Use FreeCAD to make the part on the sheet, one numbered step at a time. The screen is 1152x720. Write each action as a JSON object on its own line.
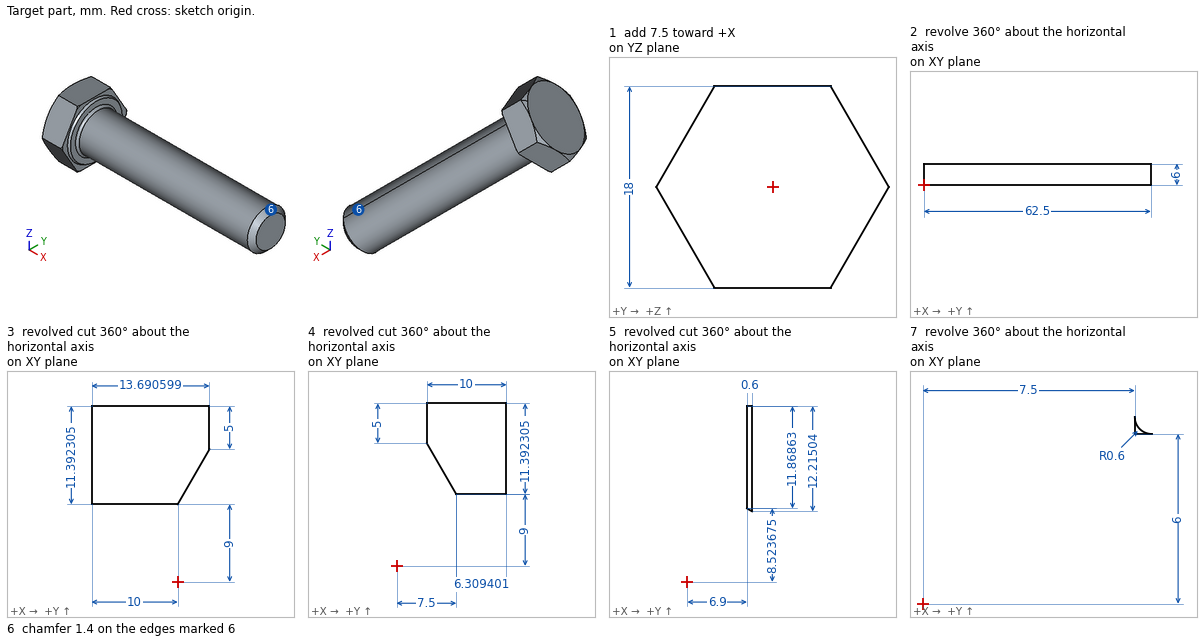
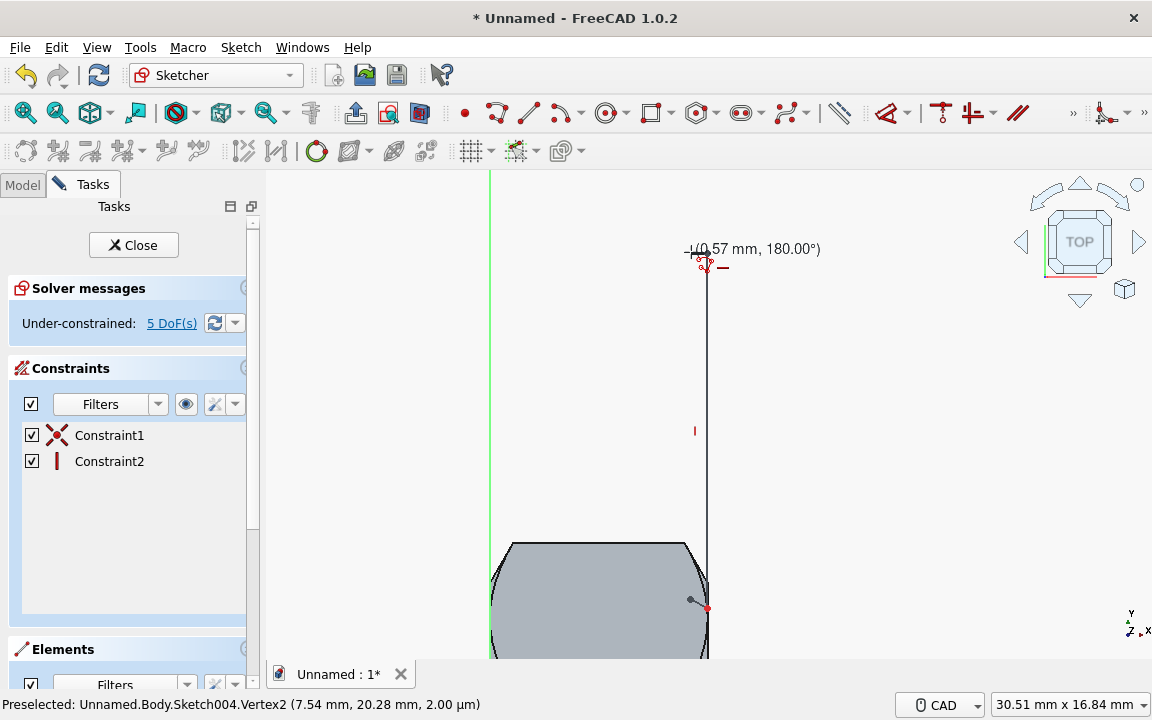
{"action": "left_click", "coordinate": [690, 252]}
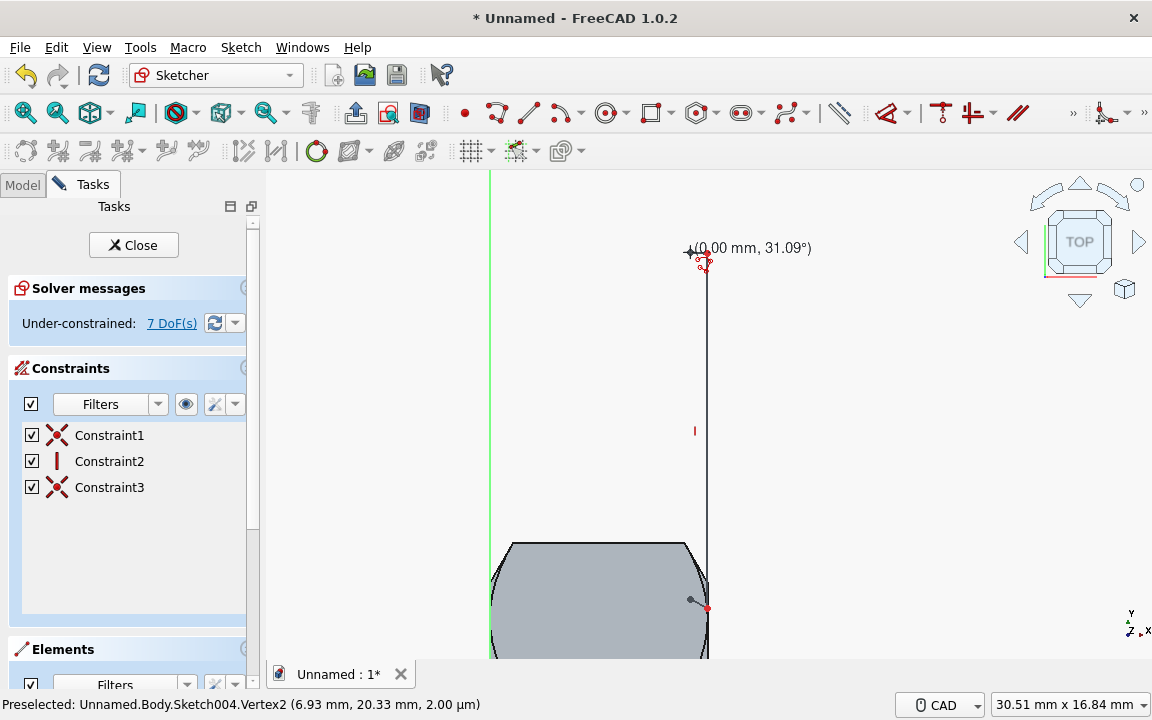
{"action": "scroll", "coordinate": [690, 597], "scroll_direction": "up", "scroll_amount": 3}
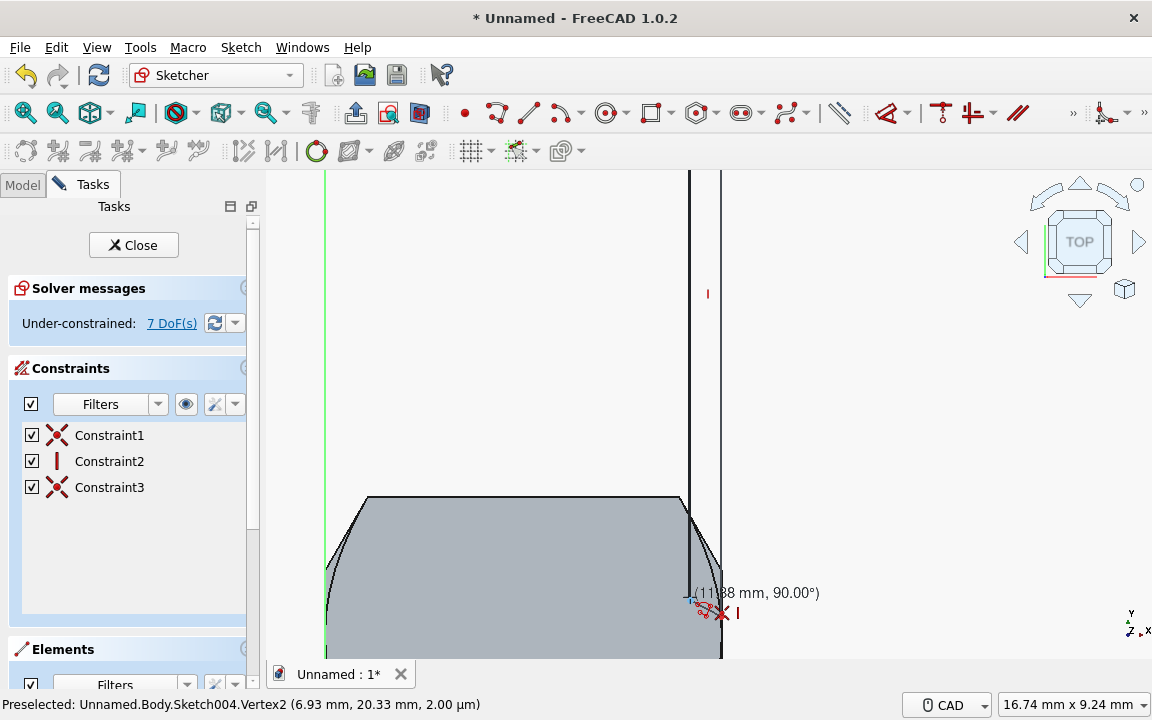
{"action": "left_click", "coordinate": [691, 600]}
{"action": "key", "text": "Escape"}
{"action": "key", "text": "Escape"}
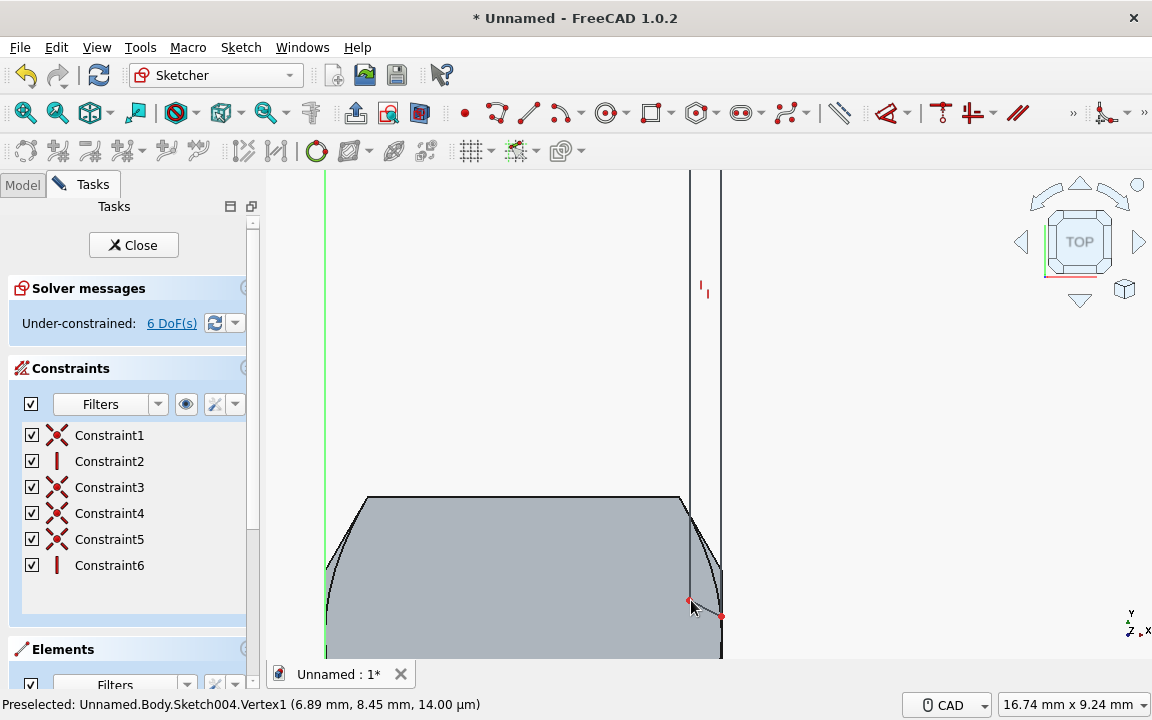
{"action": "scroll", "coordinate": [691, 374], "scroll_direction": "down", "scroll_amount": 6}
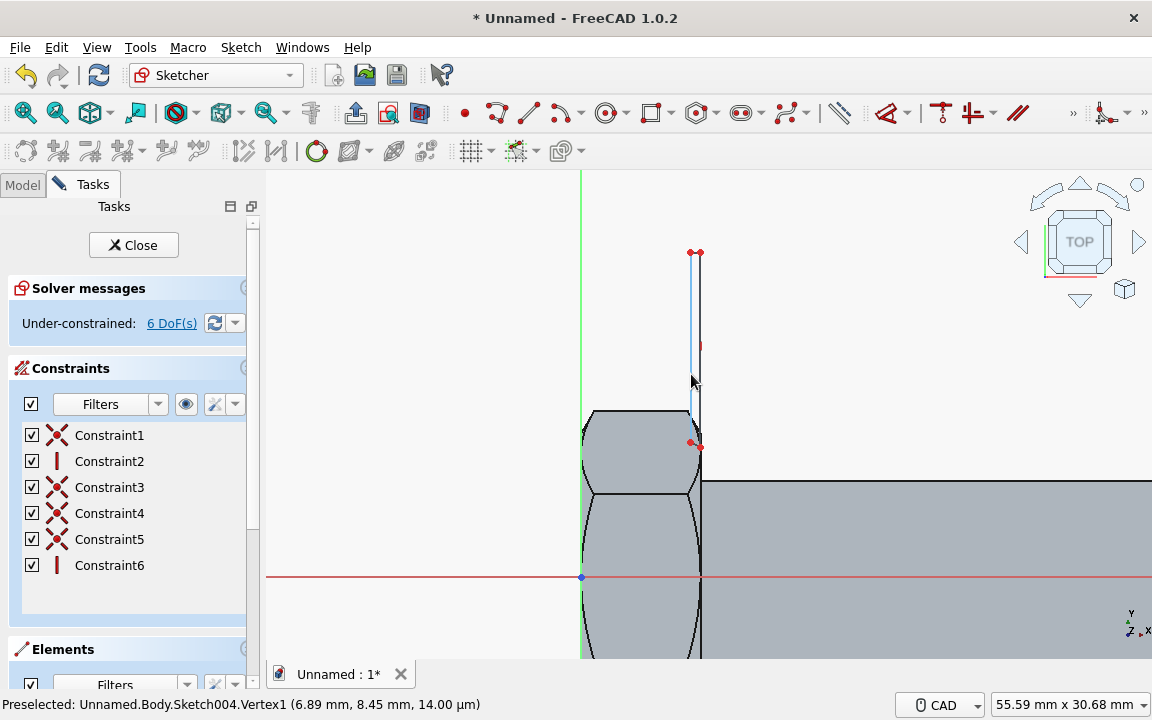
{"action": "scroll", "coordinate": [698, 253], "scroll_direction": "up", "scroll_amount": 8}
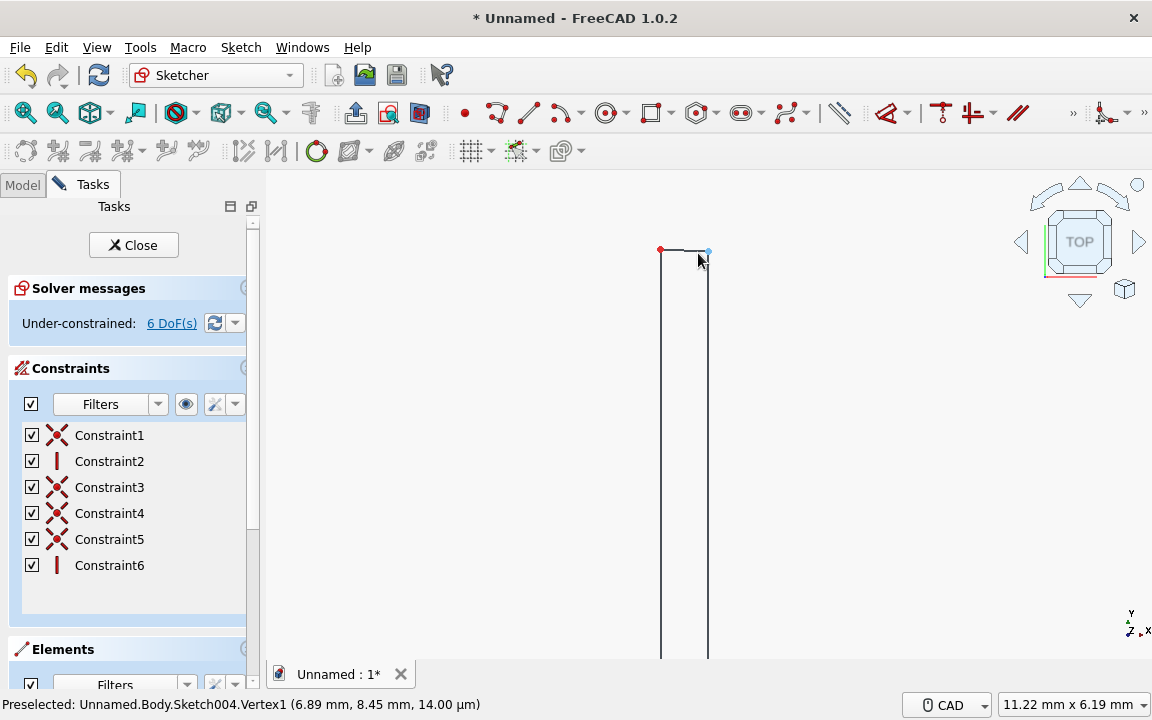
{"action": "left_click", "coordinate": [694, 251]}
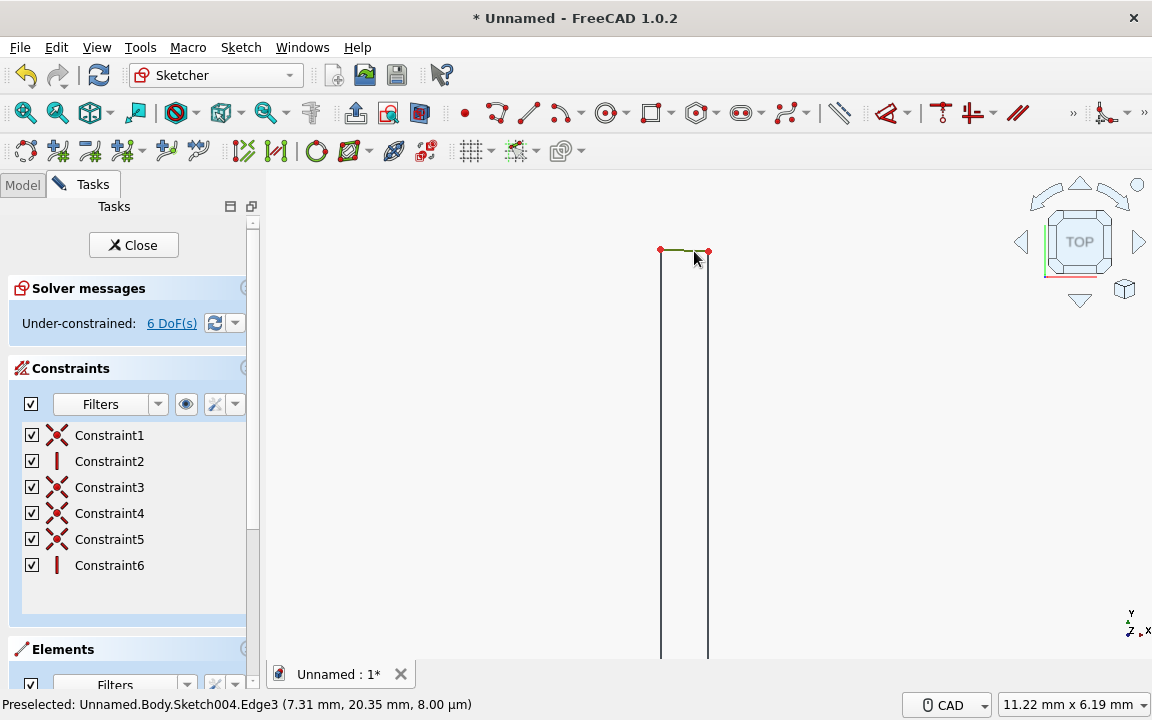
{"action": "left_click", "coordinate": [996, 114]}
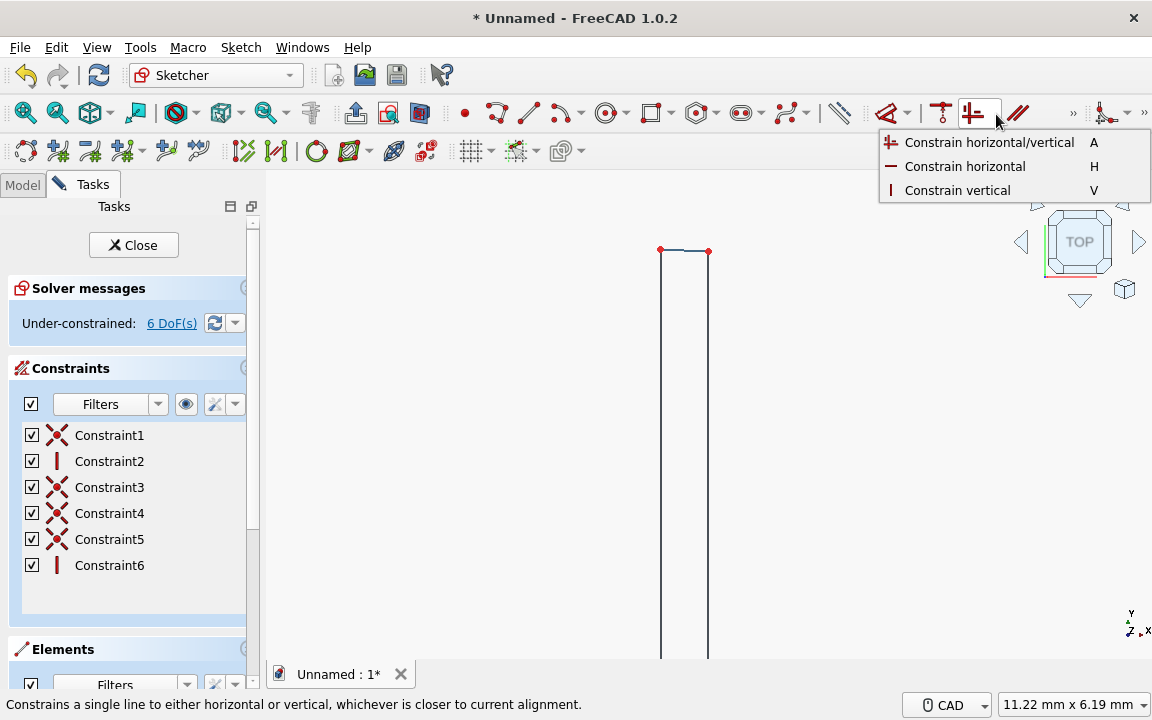
{"action": "left_click", "coordinate": [1015, 166]}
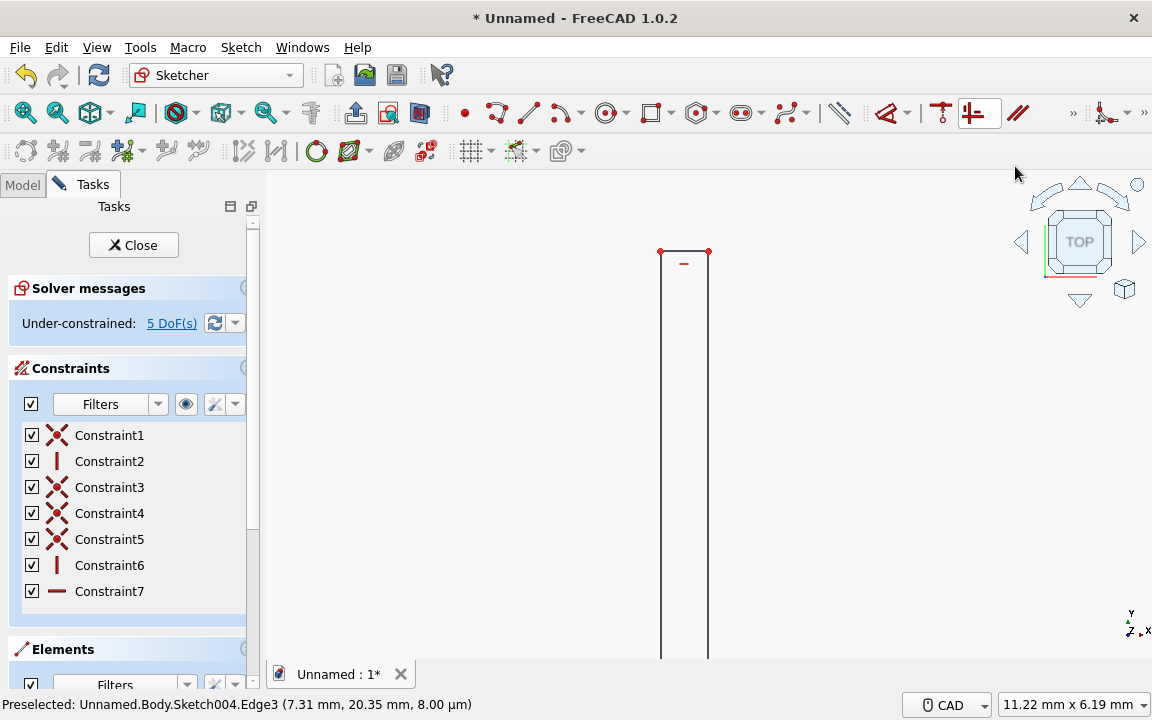
{"action": "key", "text": "d"}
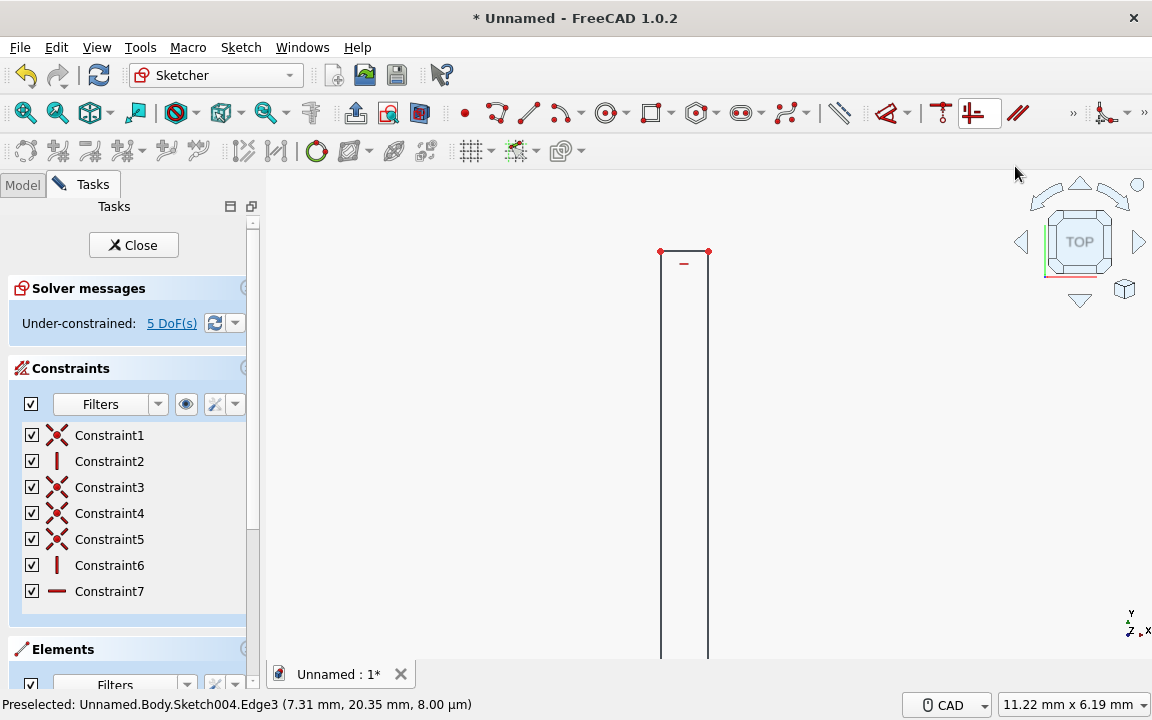
{"action": "left_click", "coordinate": [694, 251]}
{"action": "left_click", "coordinate": [684, 217]}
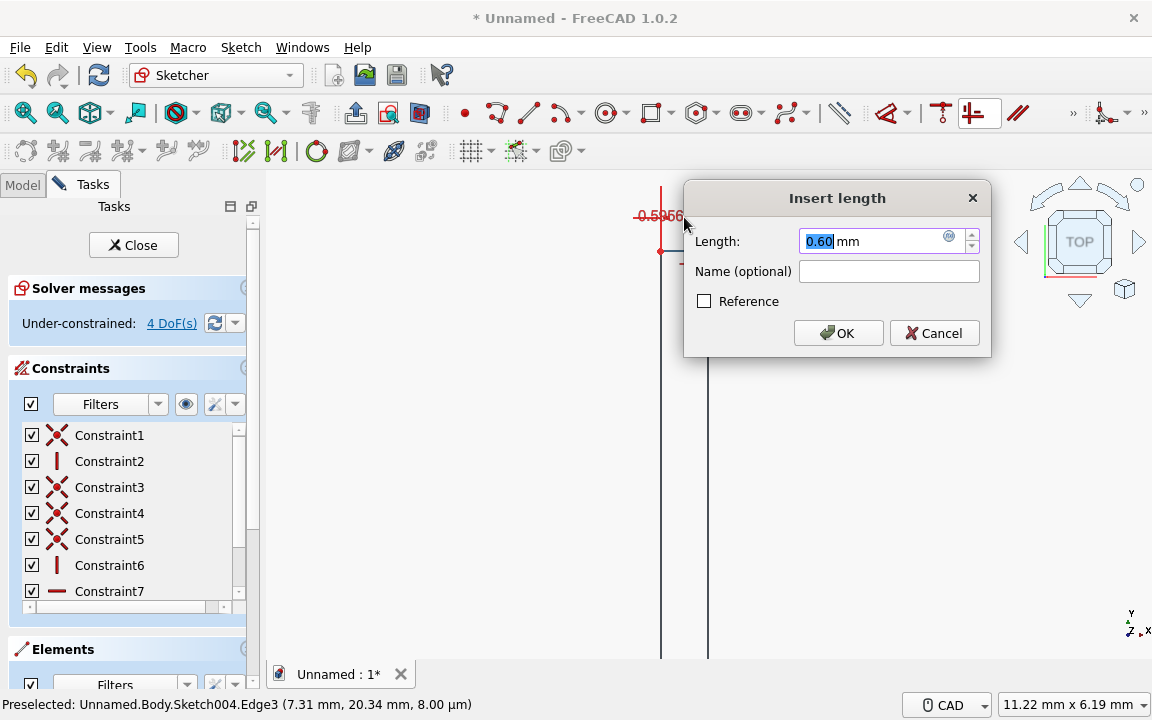
{"action": "type", "text": "0.6"}
{"action": "key", "text": "Return"}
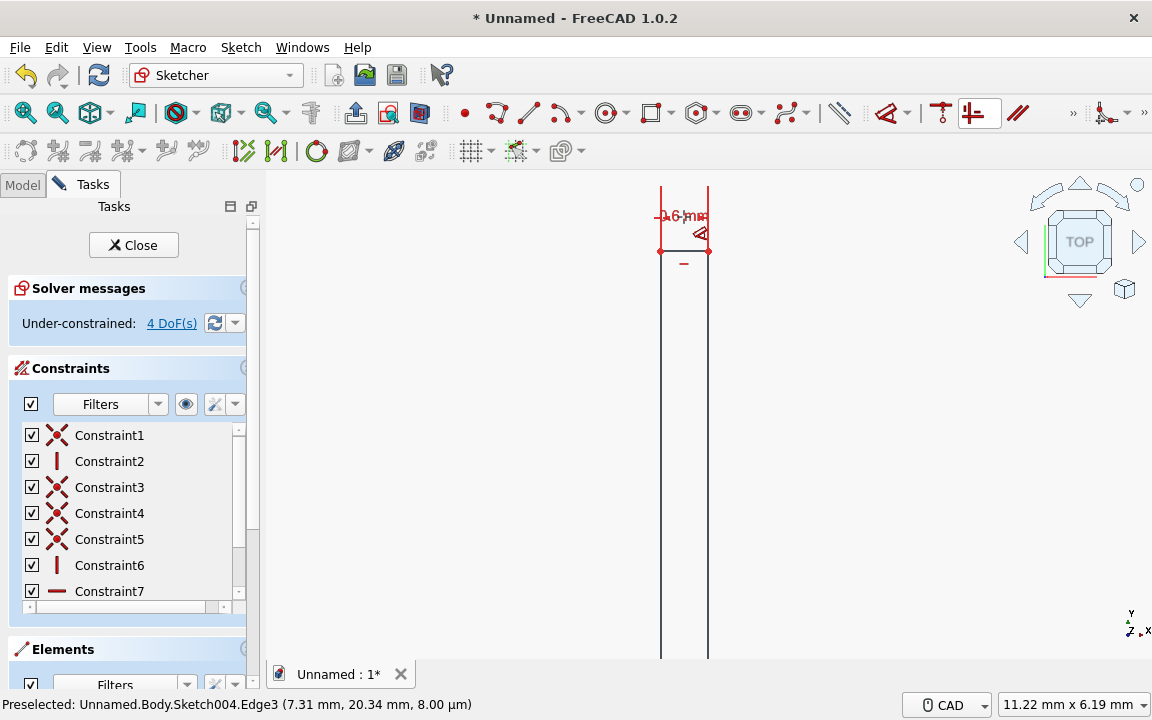
{"action": "scroll", "coordinate": [698, 253], "scroll_direction": "down", "scroll_amount": 8}